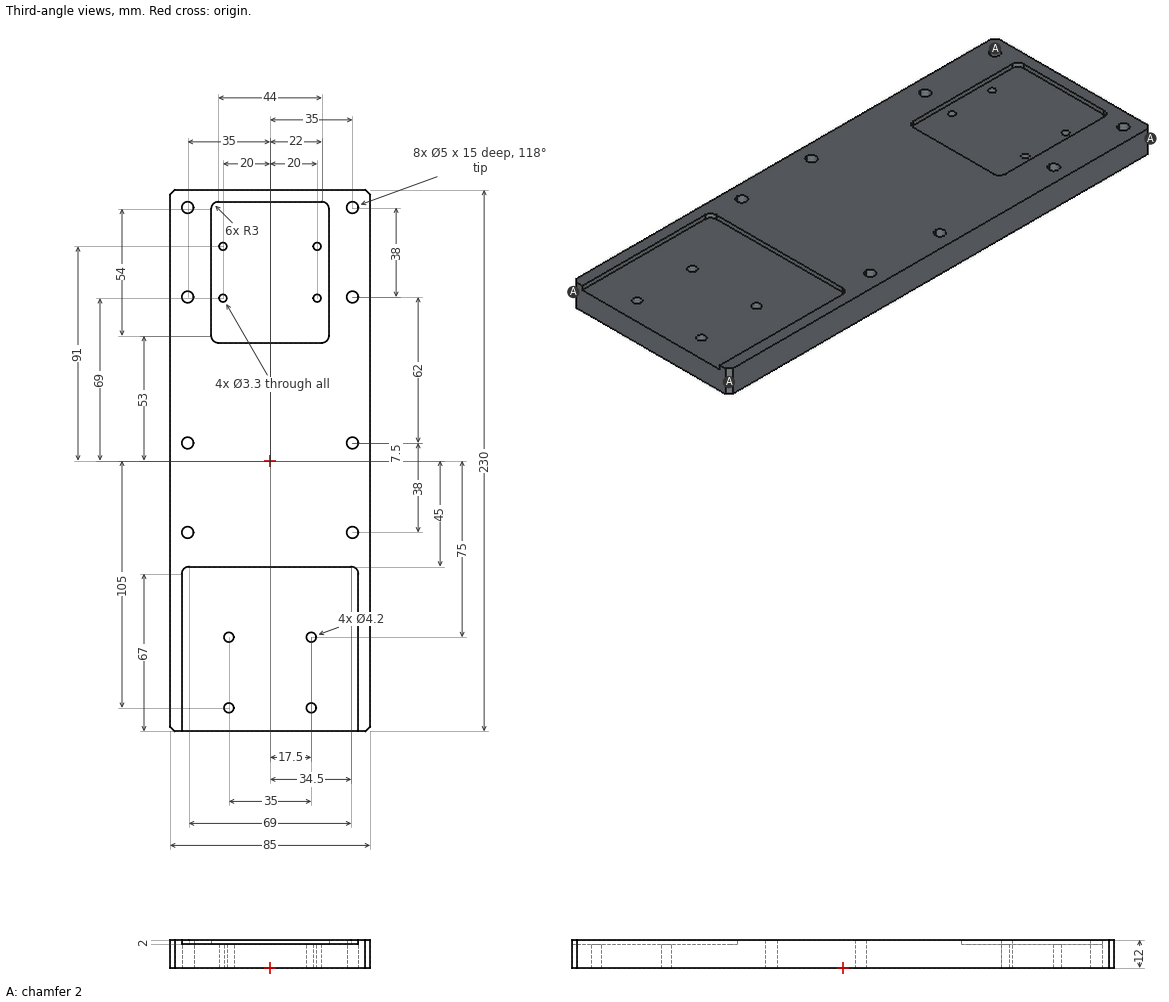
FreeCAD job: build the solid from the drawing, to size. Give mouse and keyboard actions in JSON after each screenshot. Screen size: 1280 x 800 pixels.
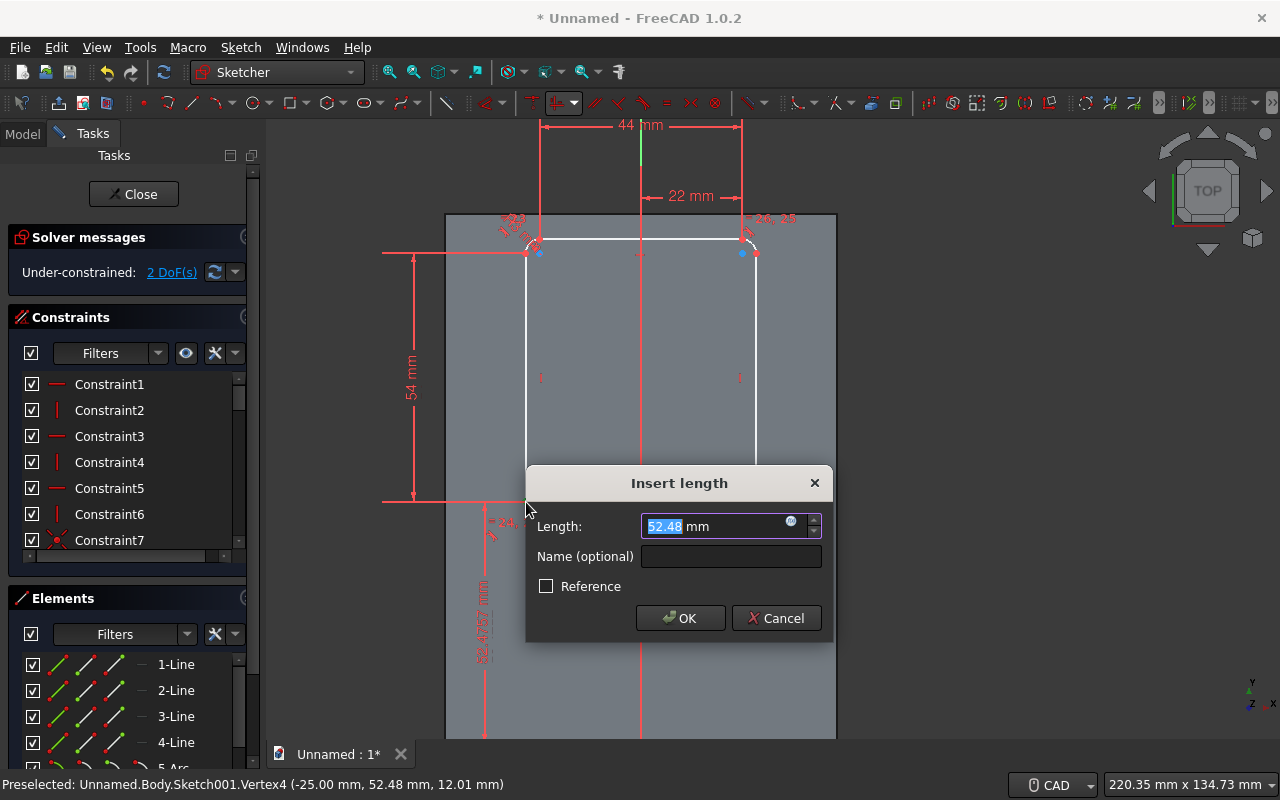
{"action": "type", "text": "53"}
{"action": "key", "text": "Return"}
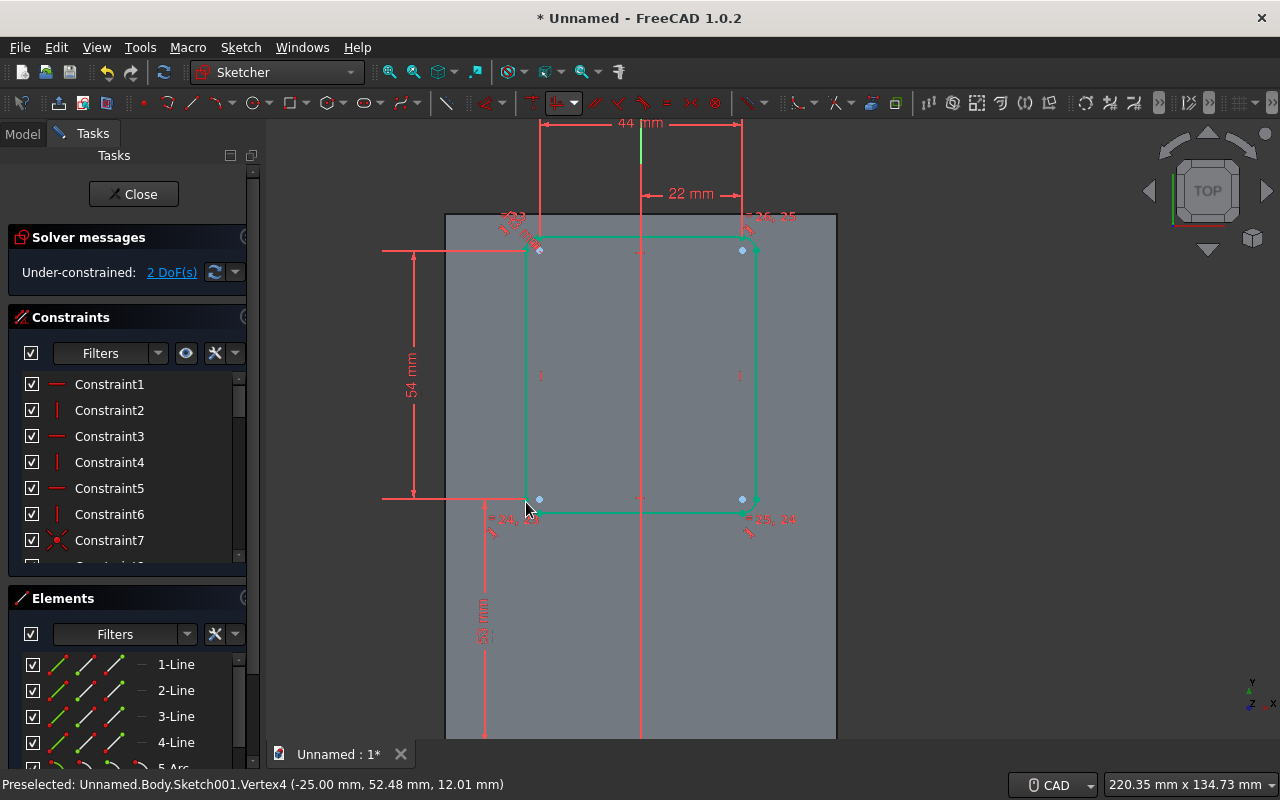
{"action": "scroll", "coordinate": [741, 239], "scroll_direction": "down", "scroll_amount": 5}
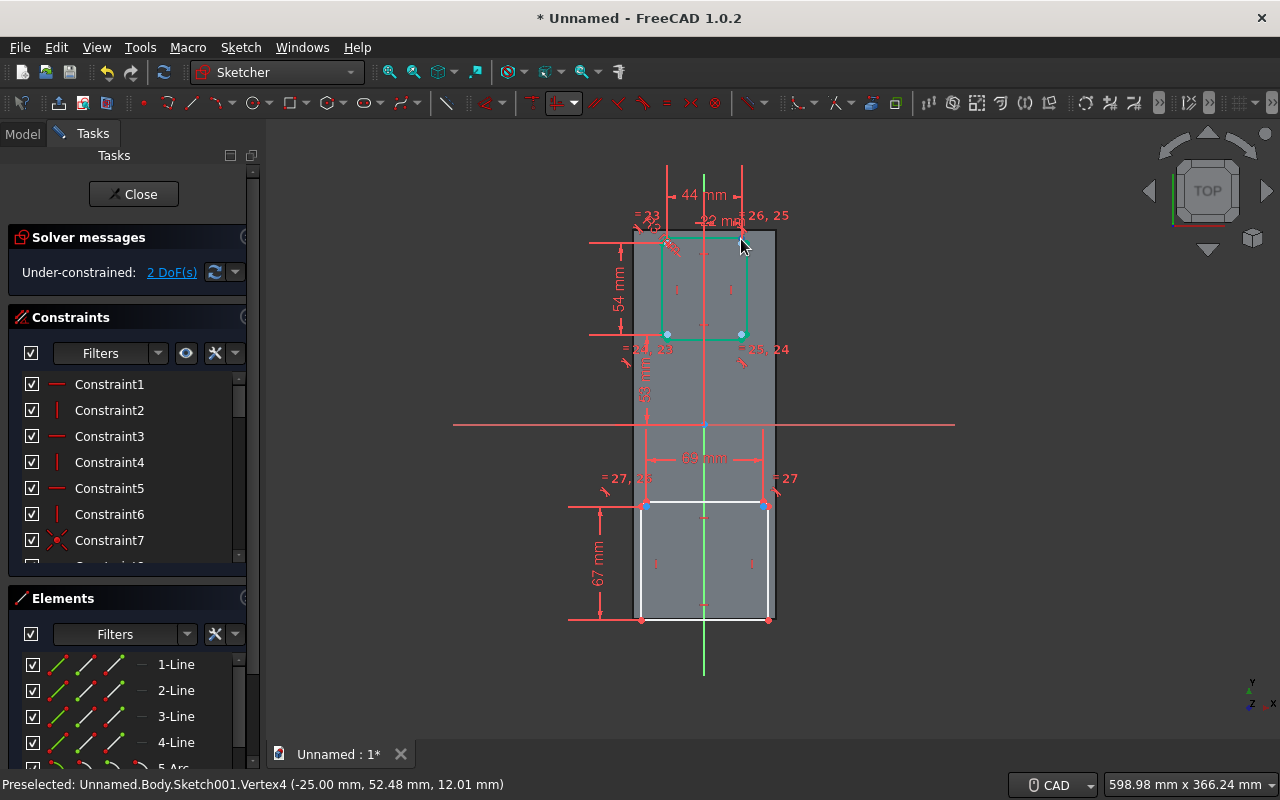
{"action": "scroll", "coordinate": [763, 502], "scroll_direction": "up", "scroll_amount": 5}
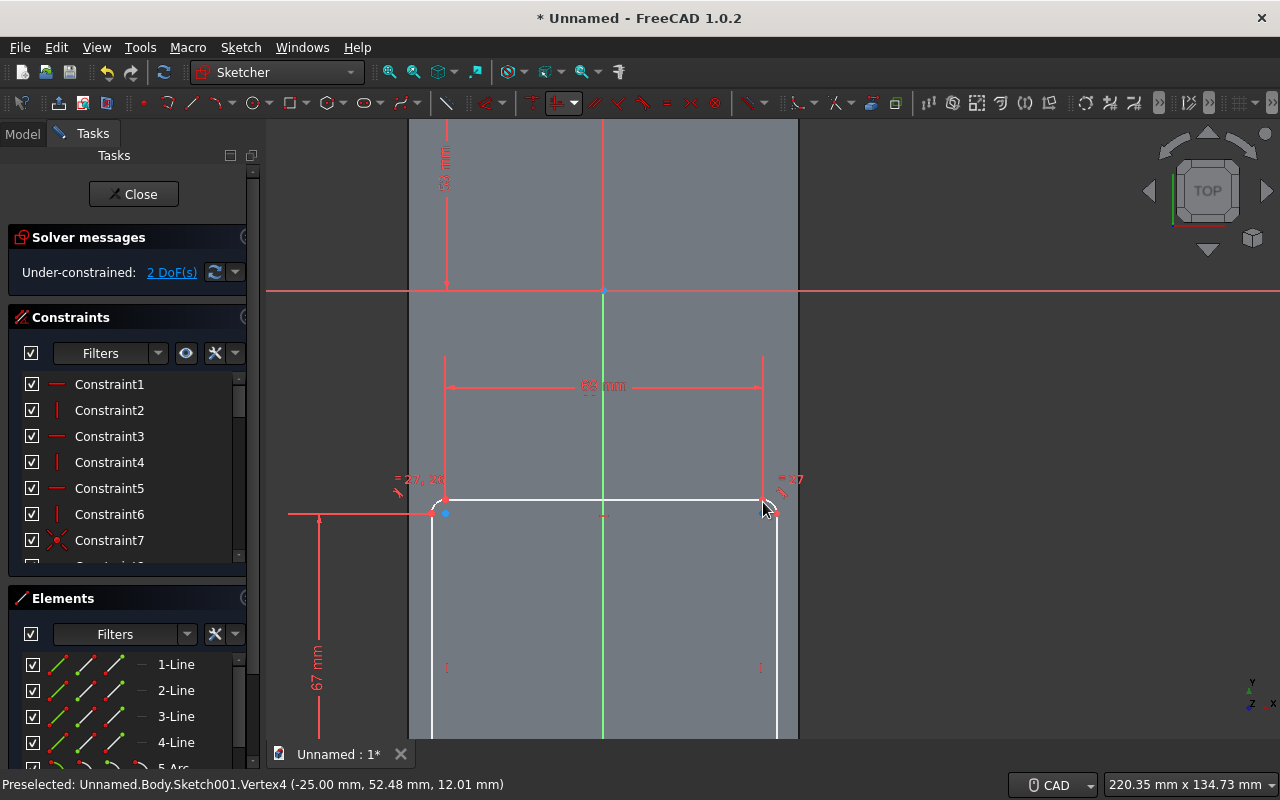
{"action": "left_click", "coordinate": [763, 500]}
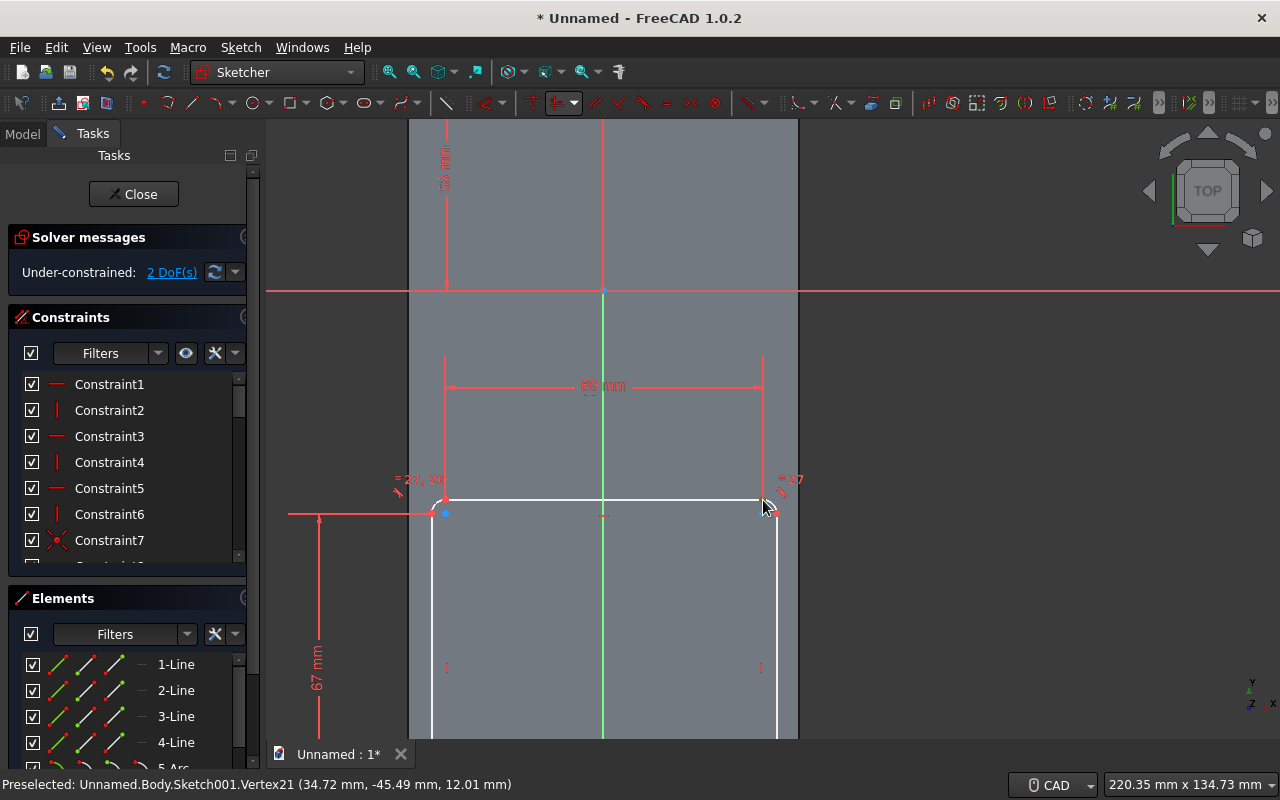
{"action": "key", "text": "i"}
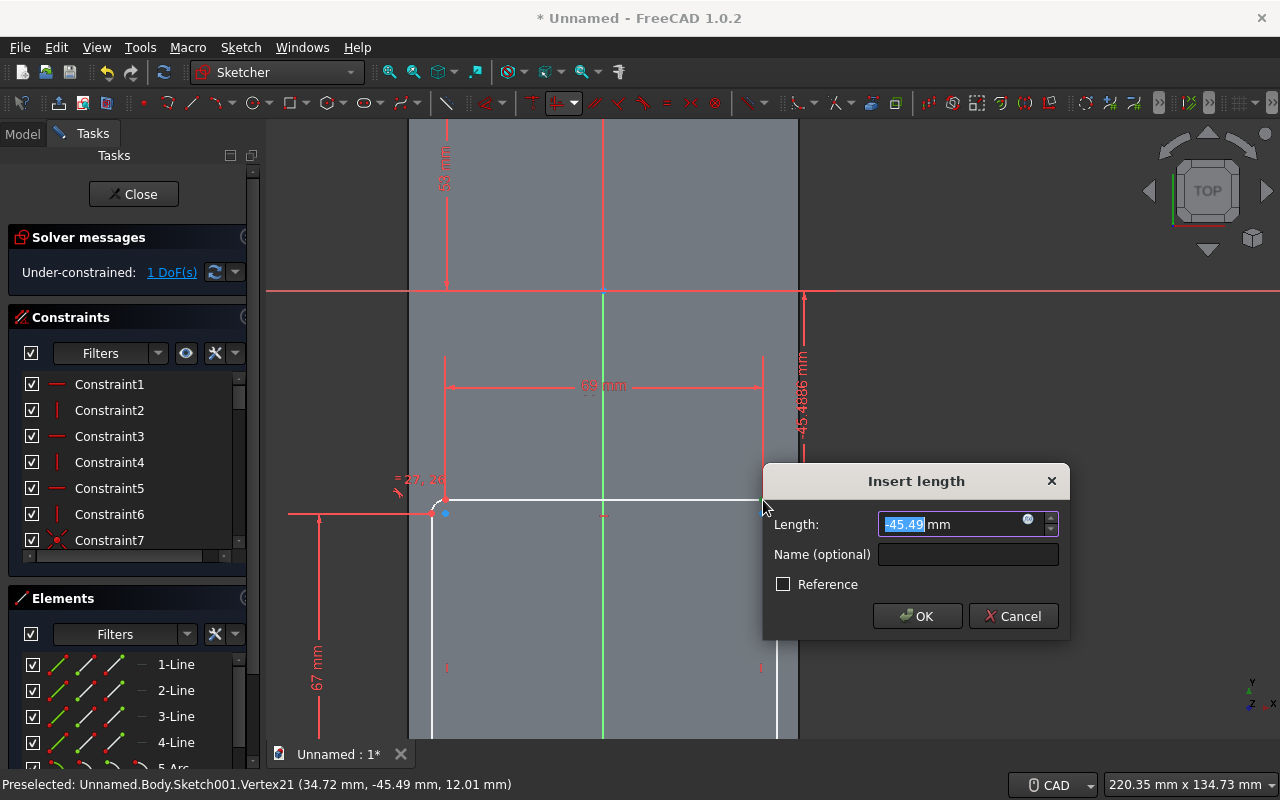
{"action": "type", "text": "-45"}
{"action": "key", "text": "Return"}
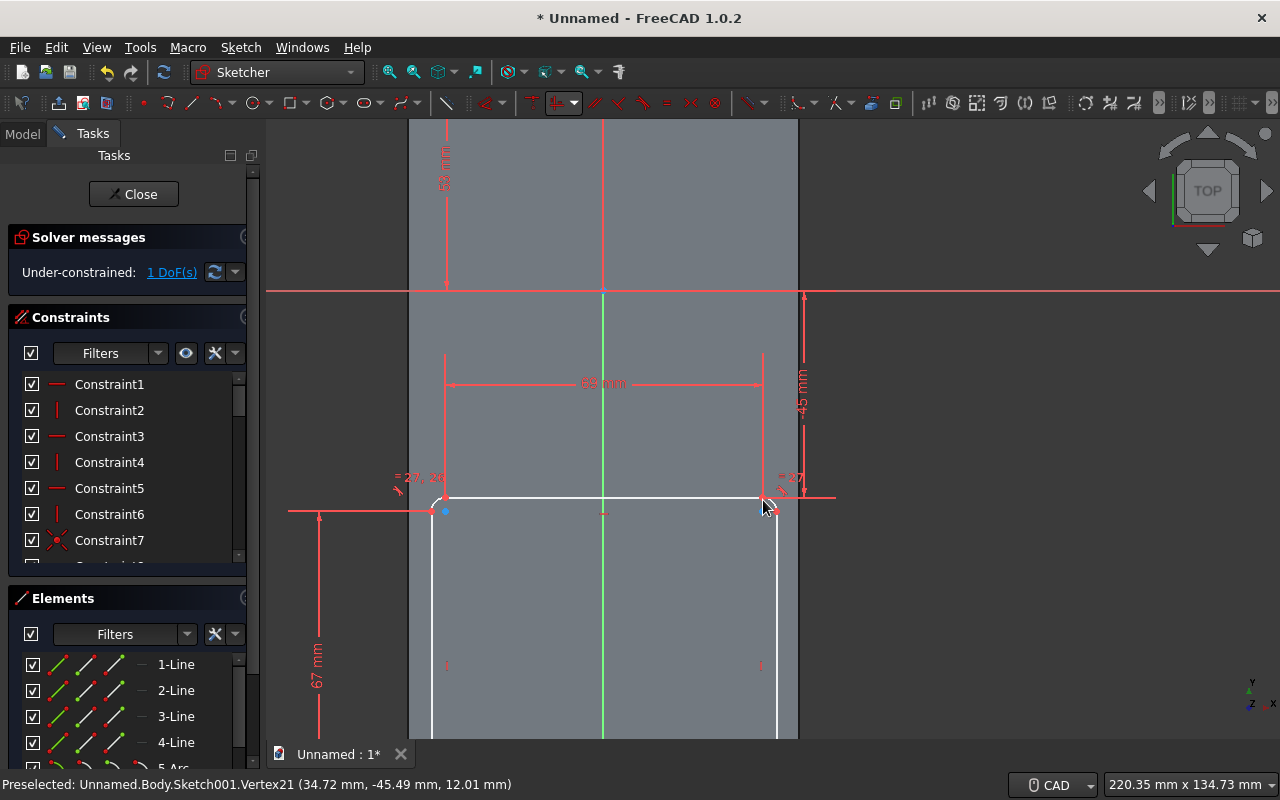
{"action": "left_click", "coordinate": [763, 498]}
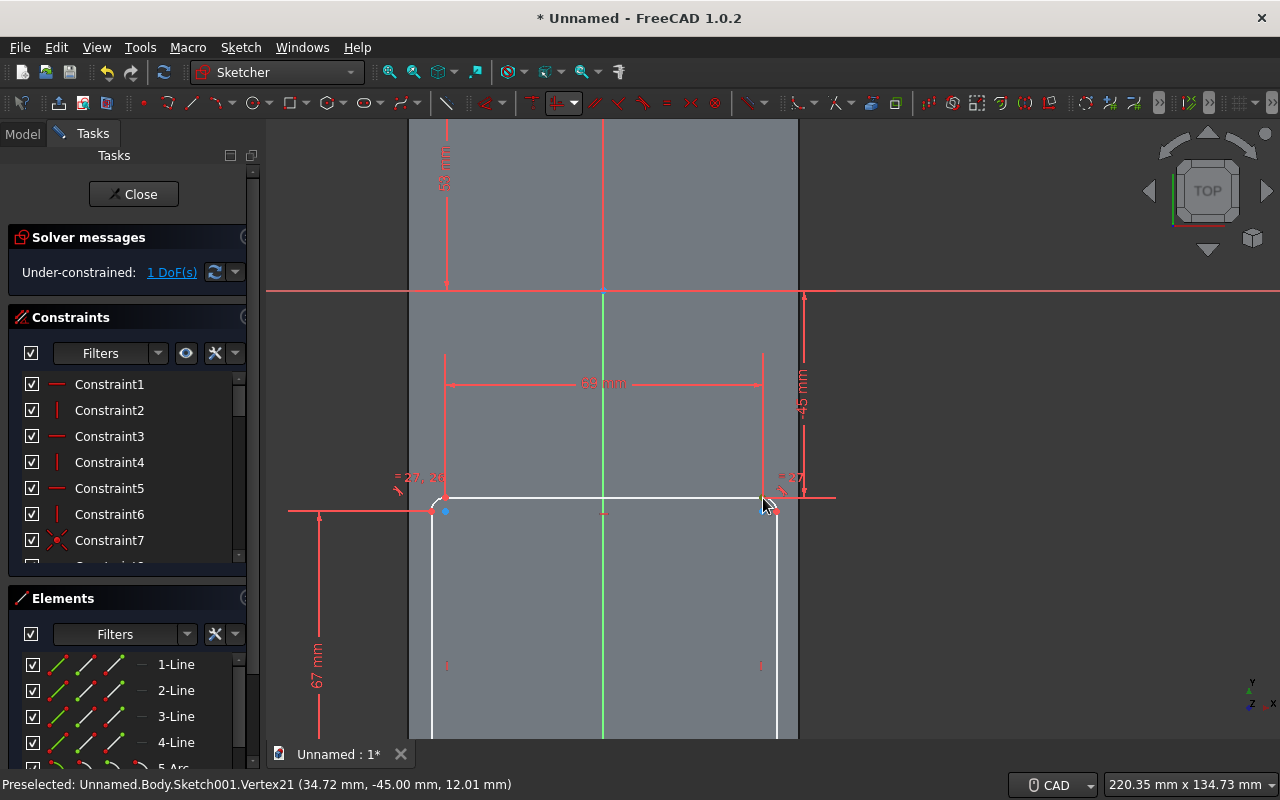
{"action": "key", "text": "l"}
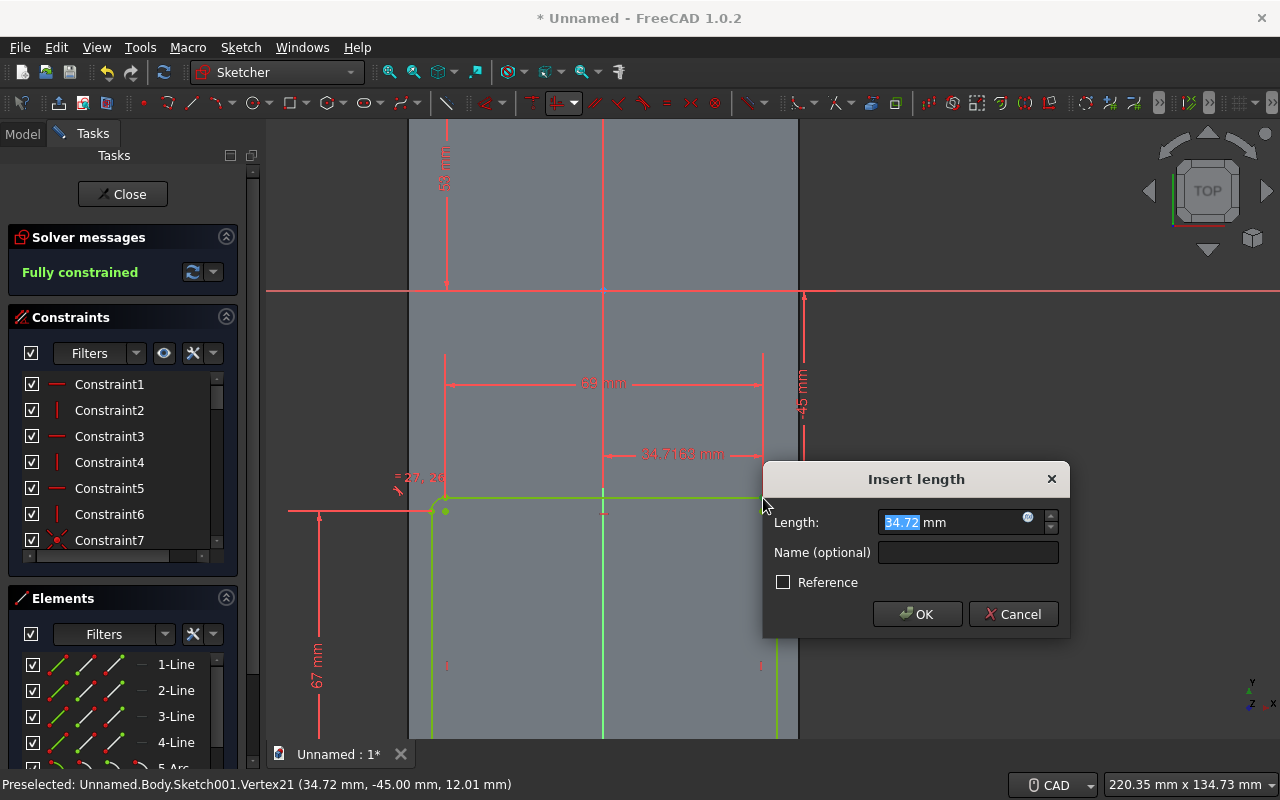
{"action": "type", "text": "34.5"}
{"action": "key", "text": "Return"}